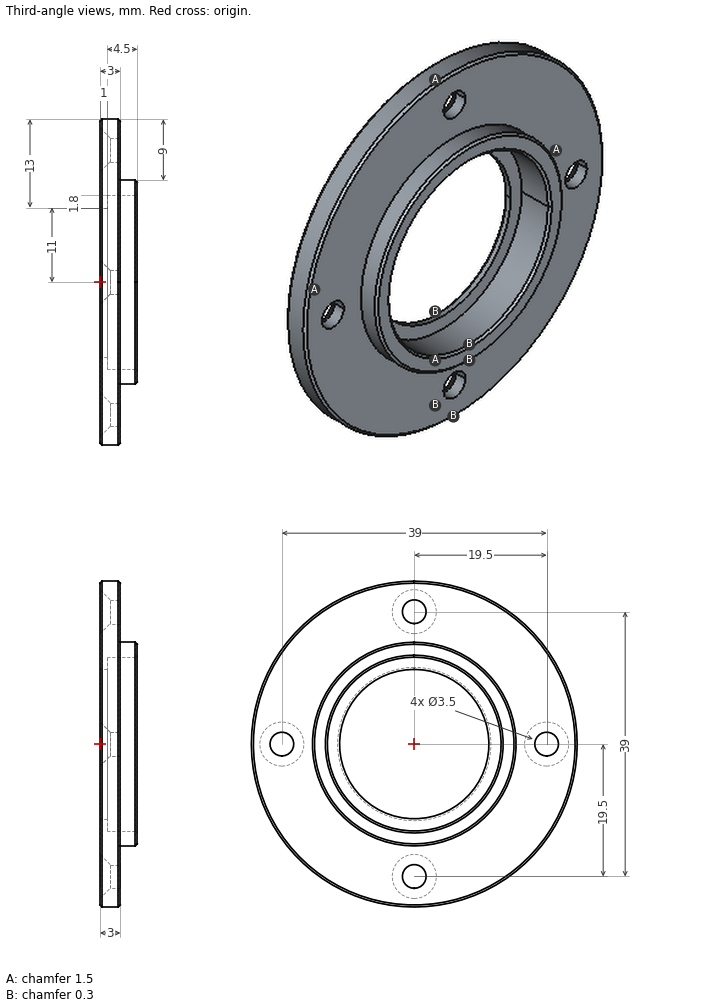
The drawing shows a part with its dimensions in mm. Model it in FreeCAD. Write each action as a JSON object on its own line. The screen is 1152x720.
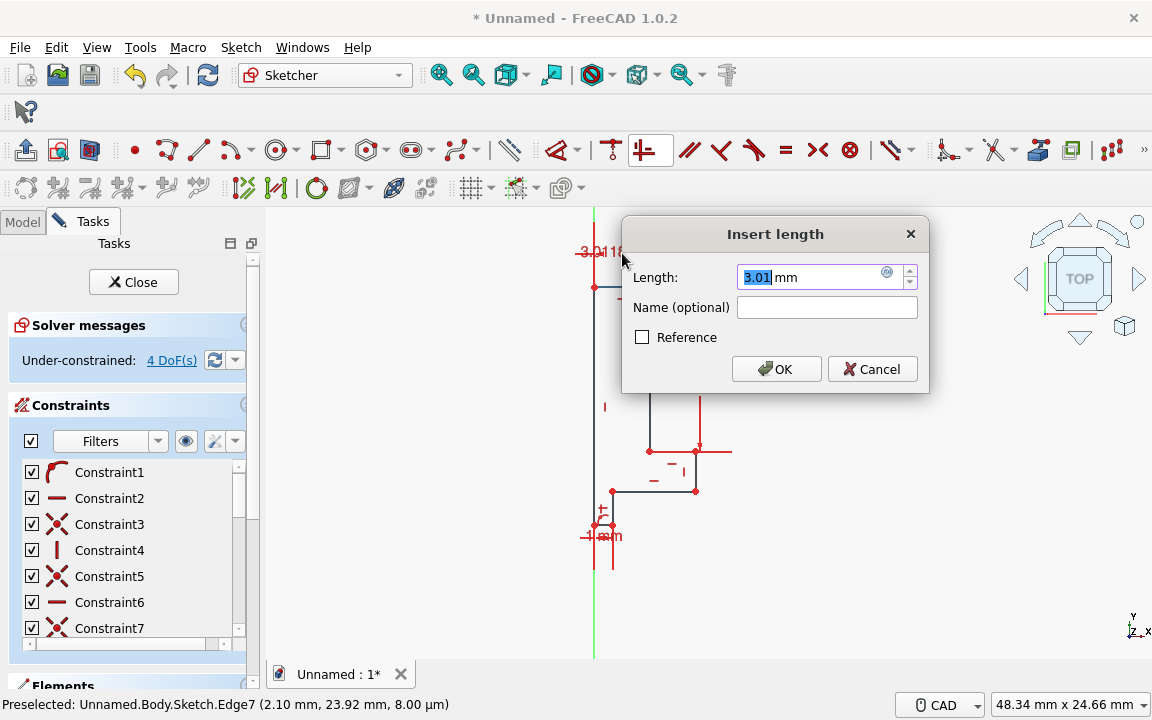
{"action": "type", "text": "3"}
{"action": "key", "text": "Return"}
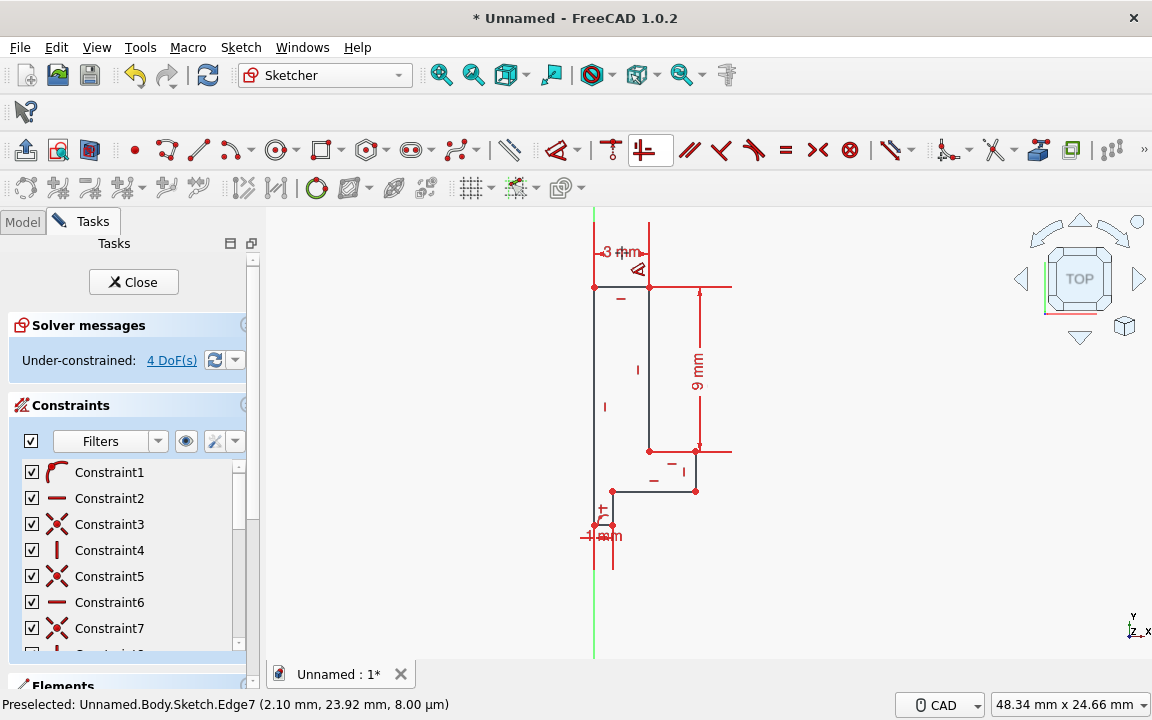
{"action": "left_click", "coordinate": [594, 358]}
{"action": "left_click", "coordinate": [560, 406]}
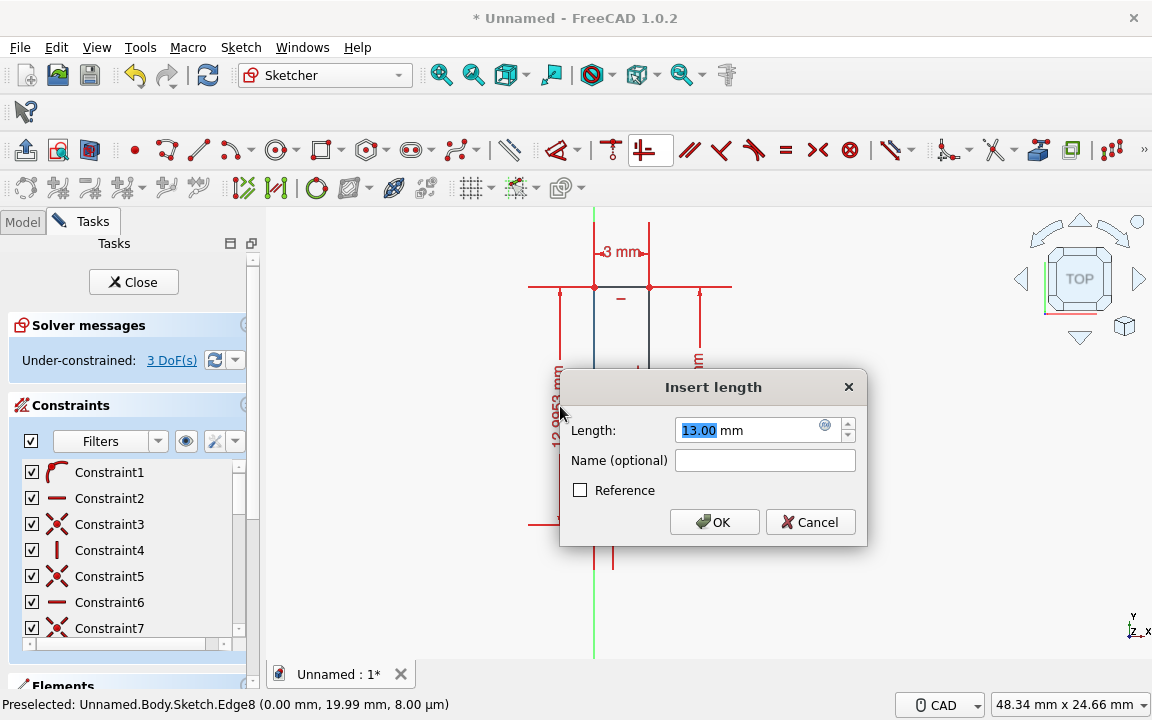
{"action": "type", "text": "13"}
{"action": "key", "text": "Return"}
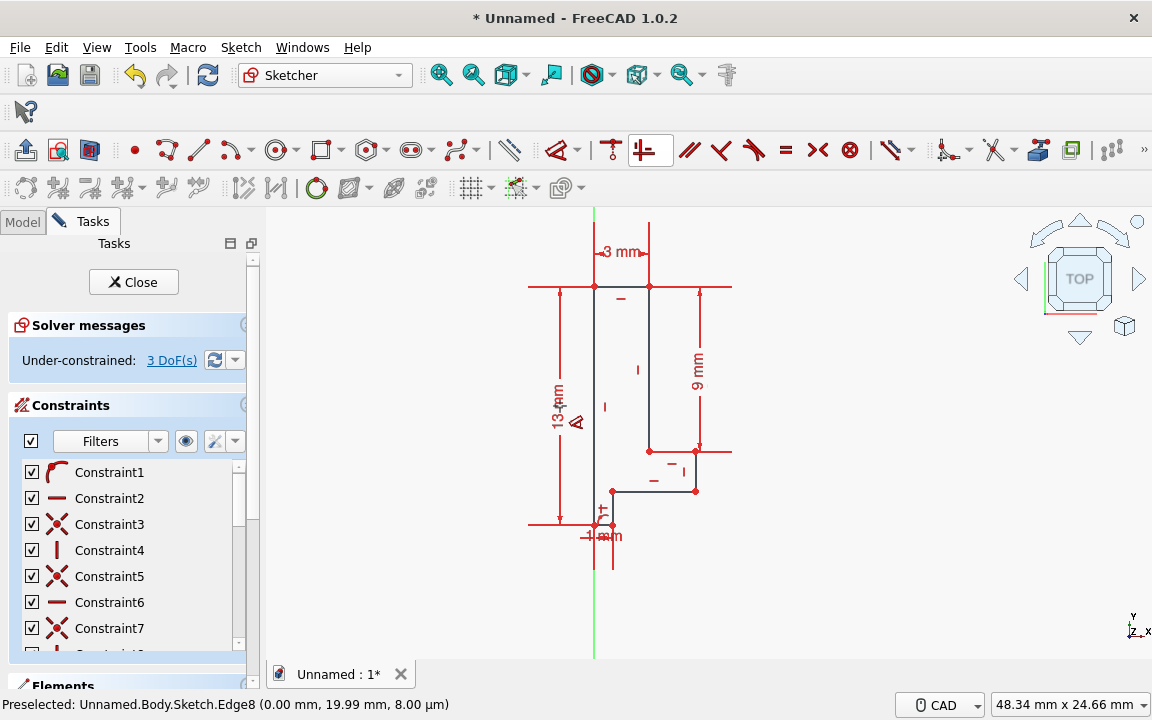
{"action": "scroll", "coordinate": [613, 515], "scroll_direction": "up", "scroll_amount": 2}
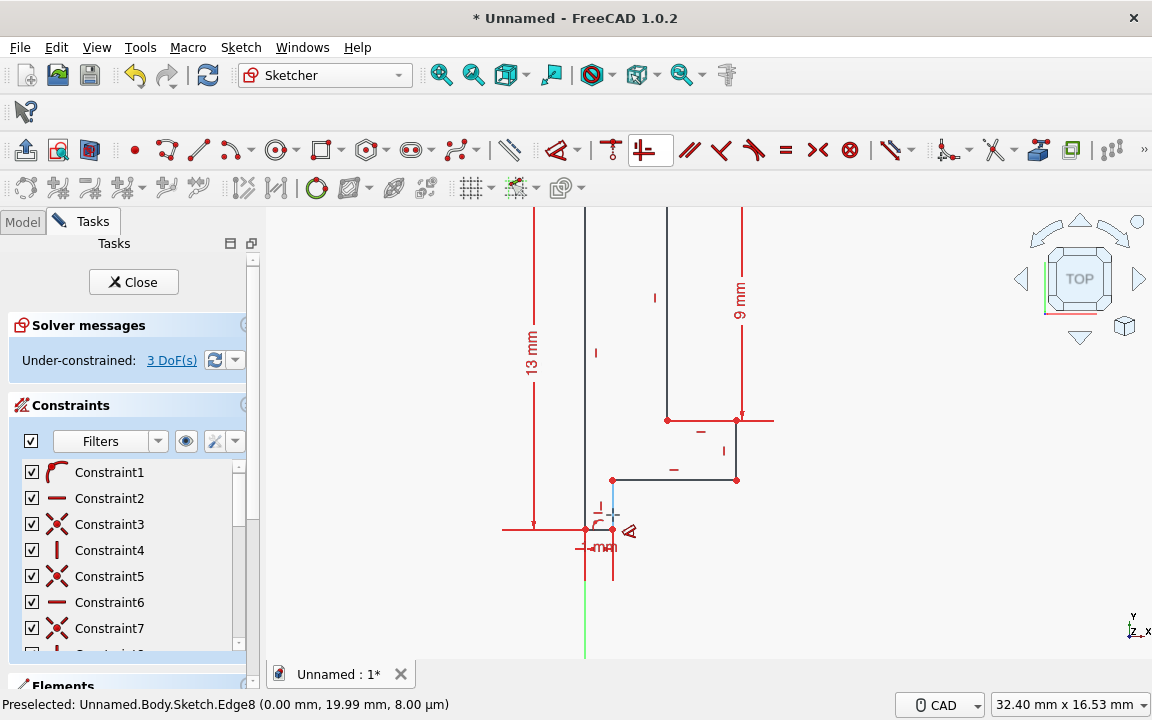
{"action": "left_click", "coordinate": [613, 515]}
{"action": "left_click", "coordinate": [647, 505]}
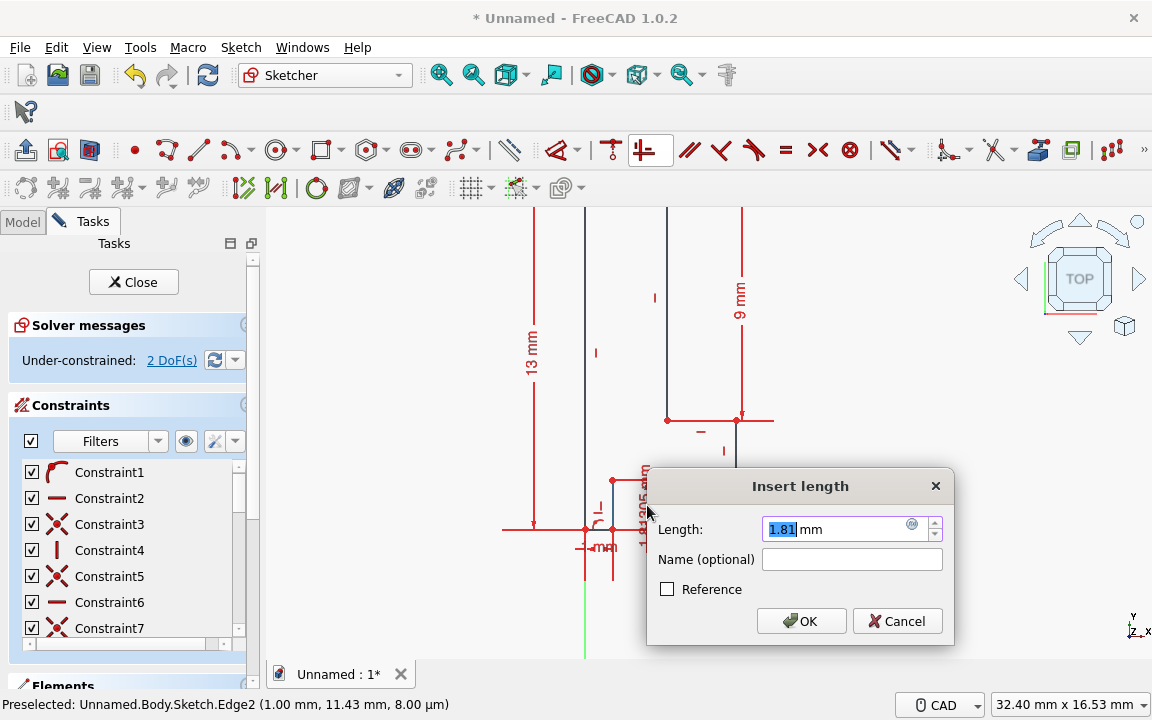
{"action": "type", "text": "1.8"}
{"action": "key", "text": "Return"}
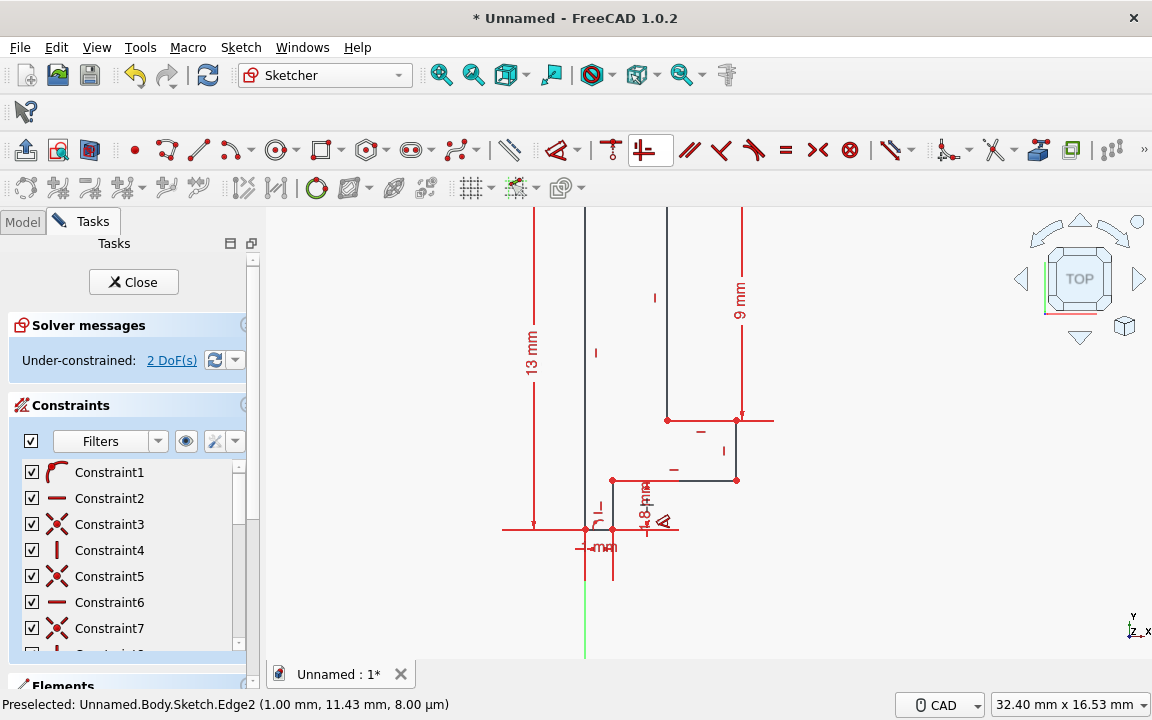
{"action": "left_click", "coordinate": [650, 481]}
{"action": "left_click", "coordinate": [674, 447]}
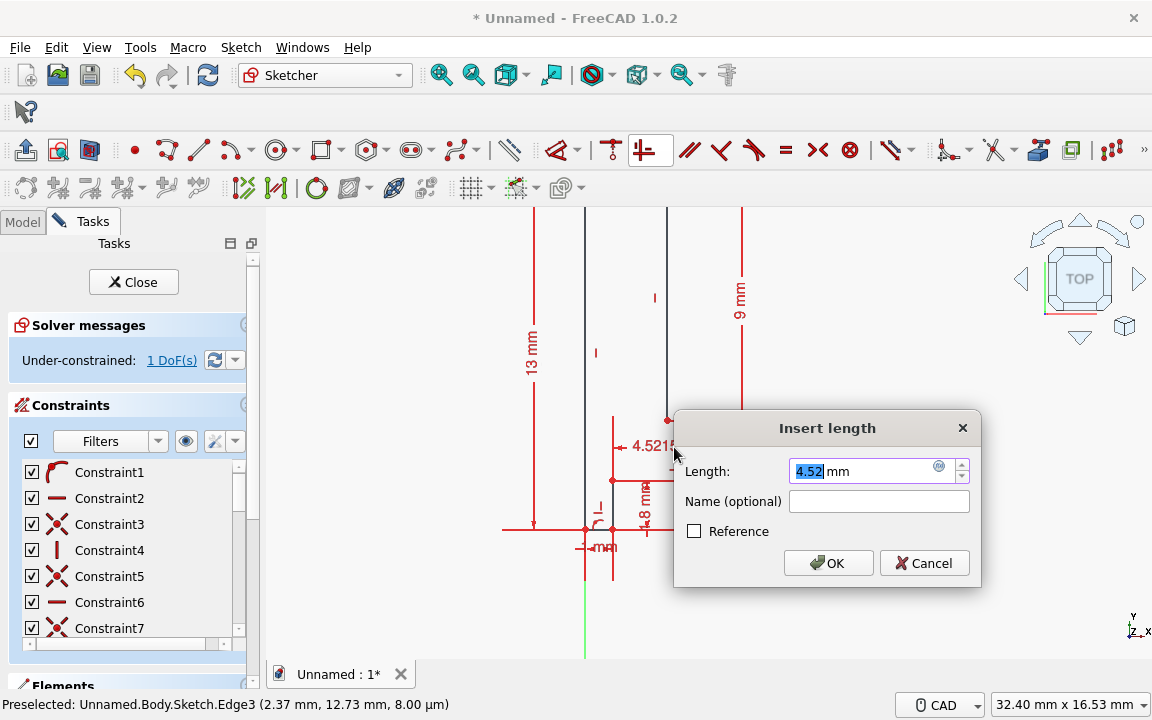
{"action": "type", "text": "4.5"}
{"action": "key", "text": "Return"}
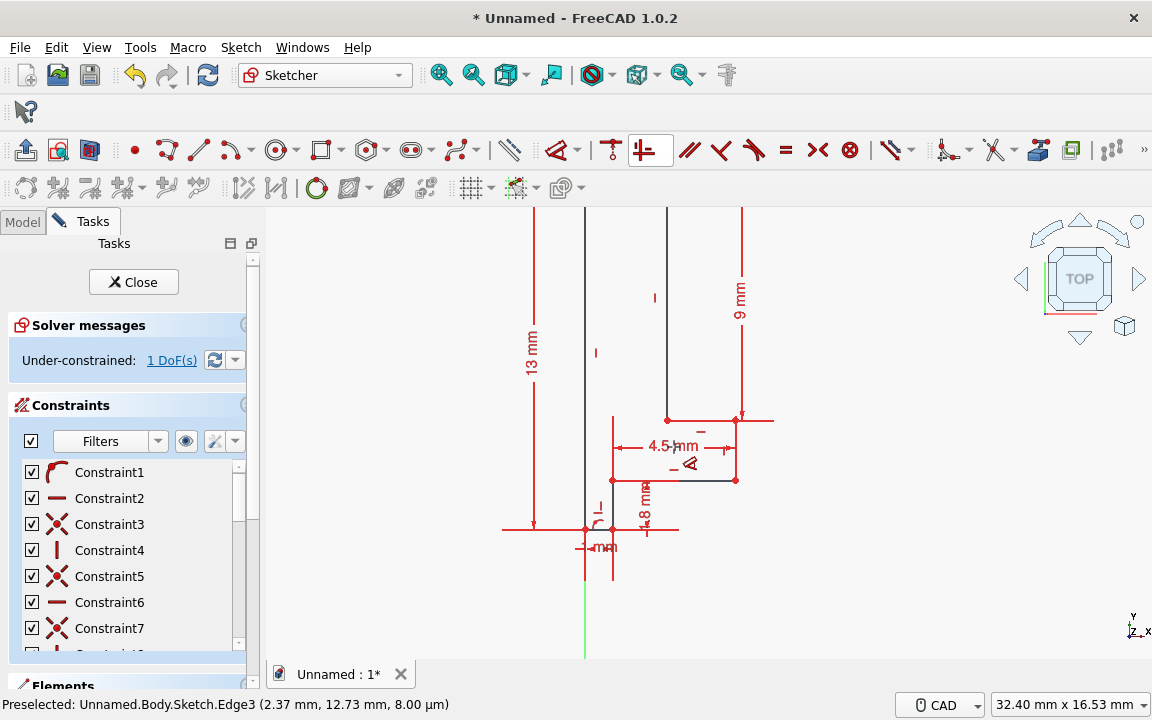
{"action": "left_click", "coordinate": [585, 530]}
{"action": "left_click", "coordinate": [551, 580]}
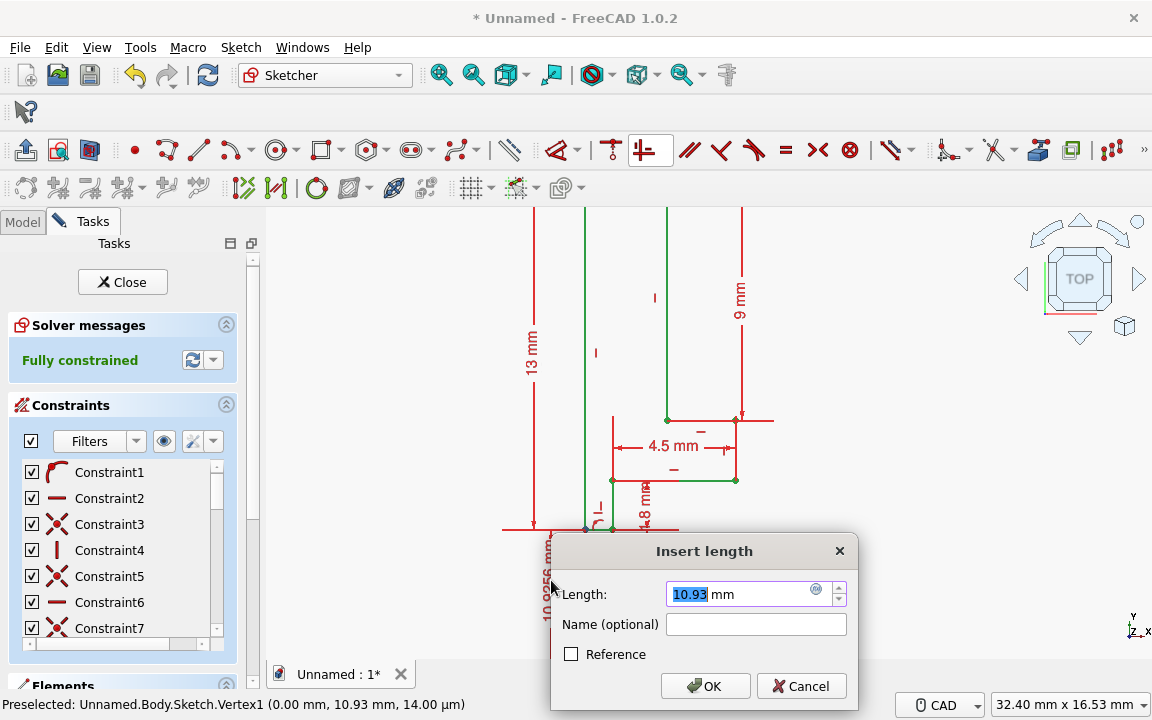
{"action": "type", "text": "11"}
{"action": "key", "text": "Return"}
{"action": "key", "text": "Escape"}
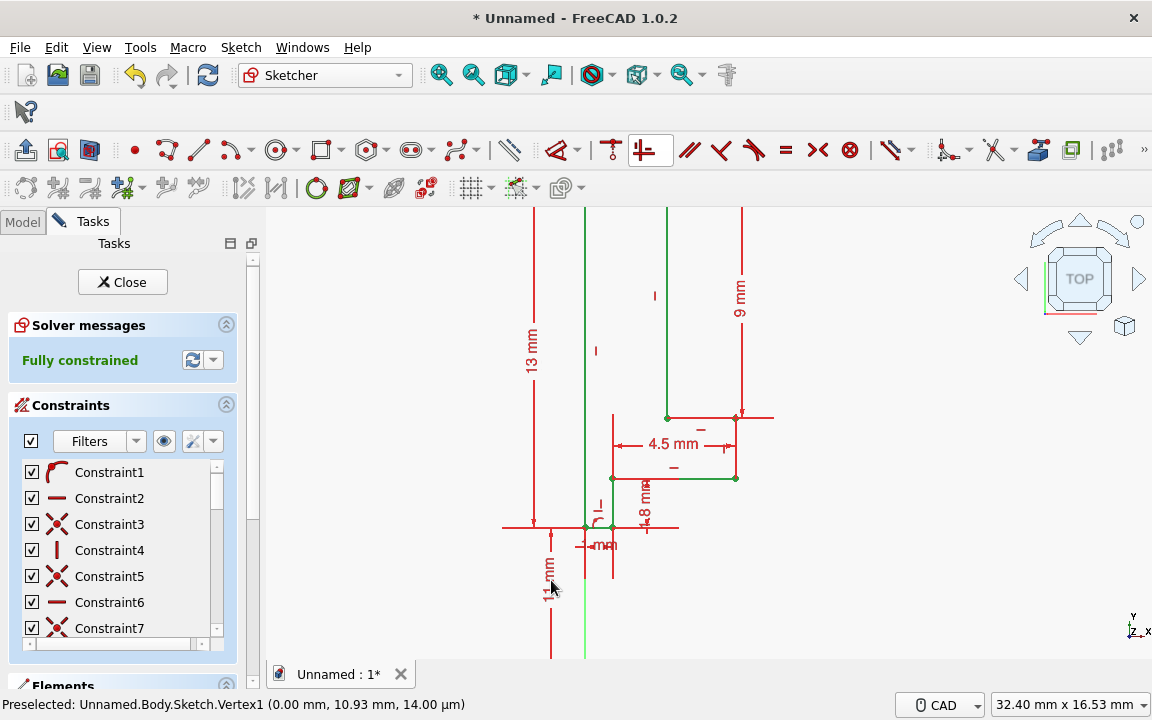
{"action": "left_click", "coordinate": [123, 282]}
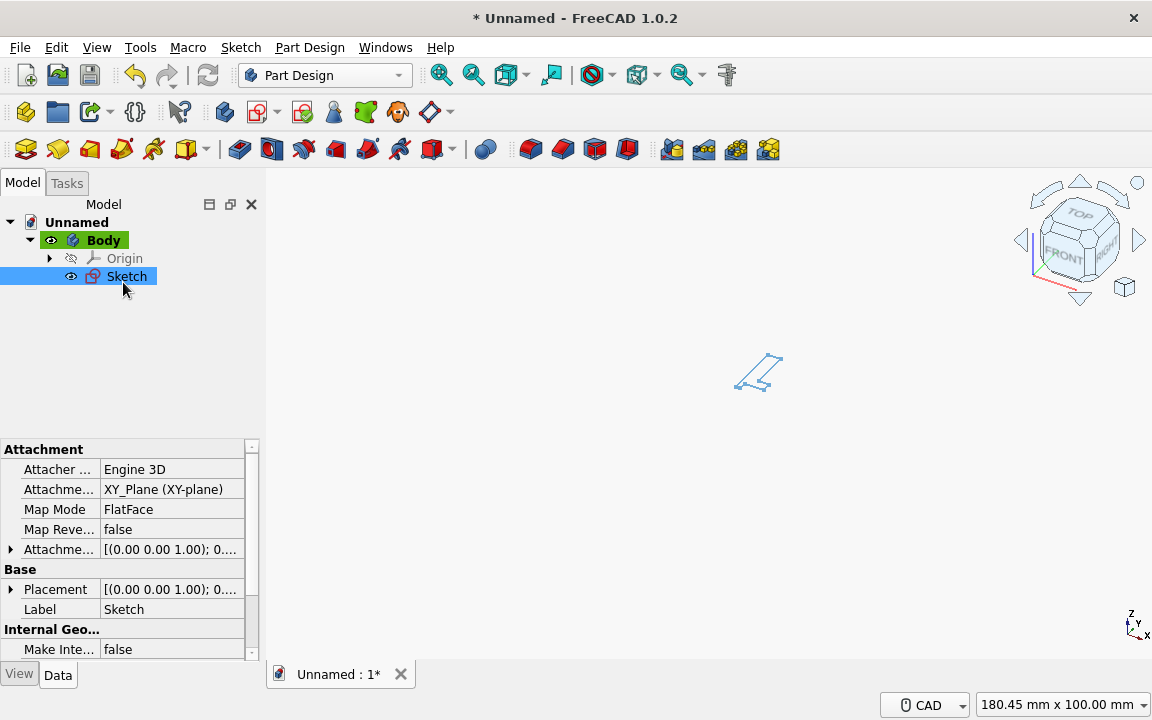
{"action": "left_click", "coordinate": [58, 150]}